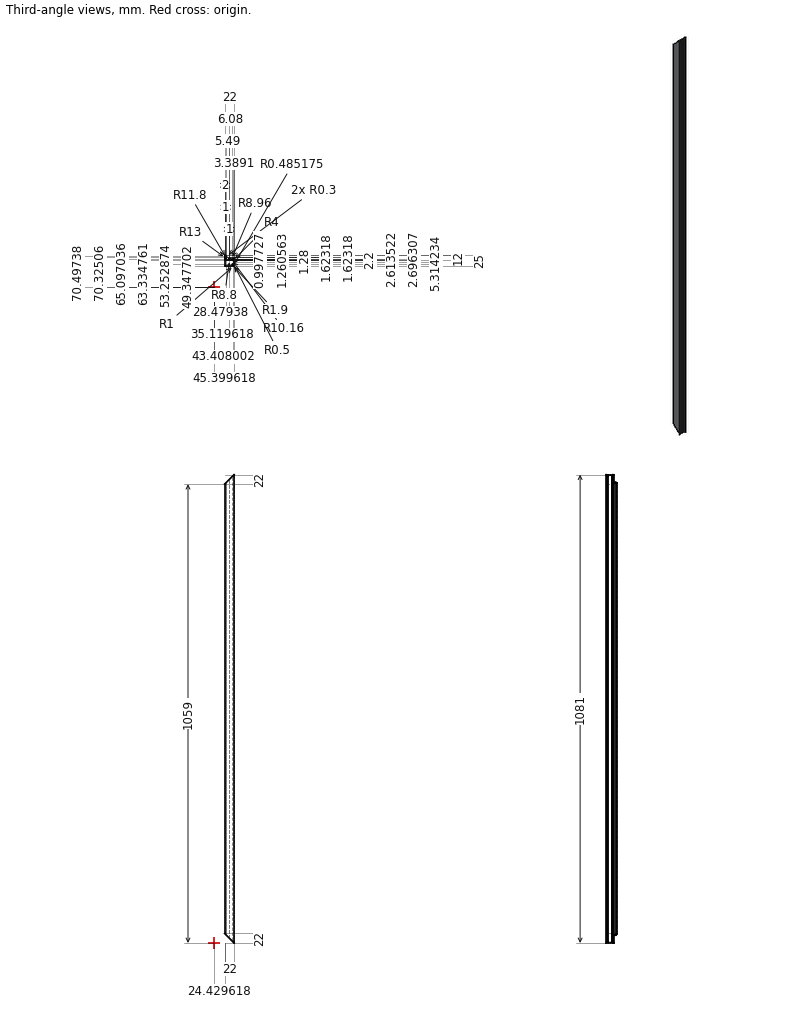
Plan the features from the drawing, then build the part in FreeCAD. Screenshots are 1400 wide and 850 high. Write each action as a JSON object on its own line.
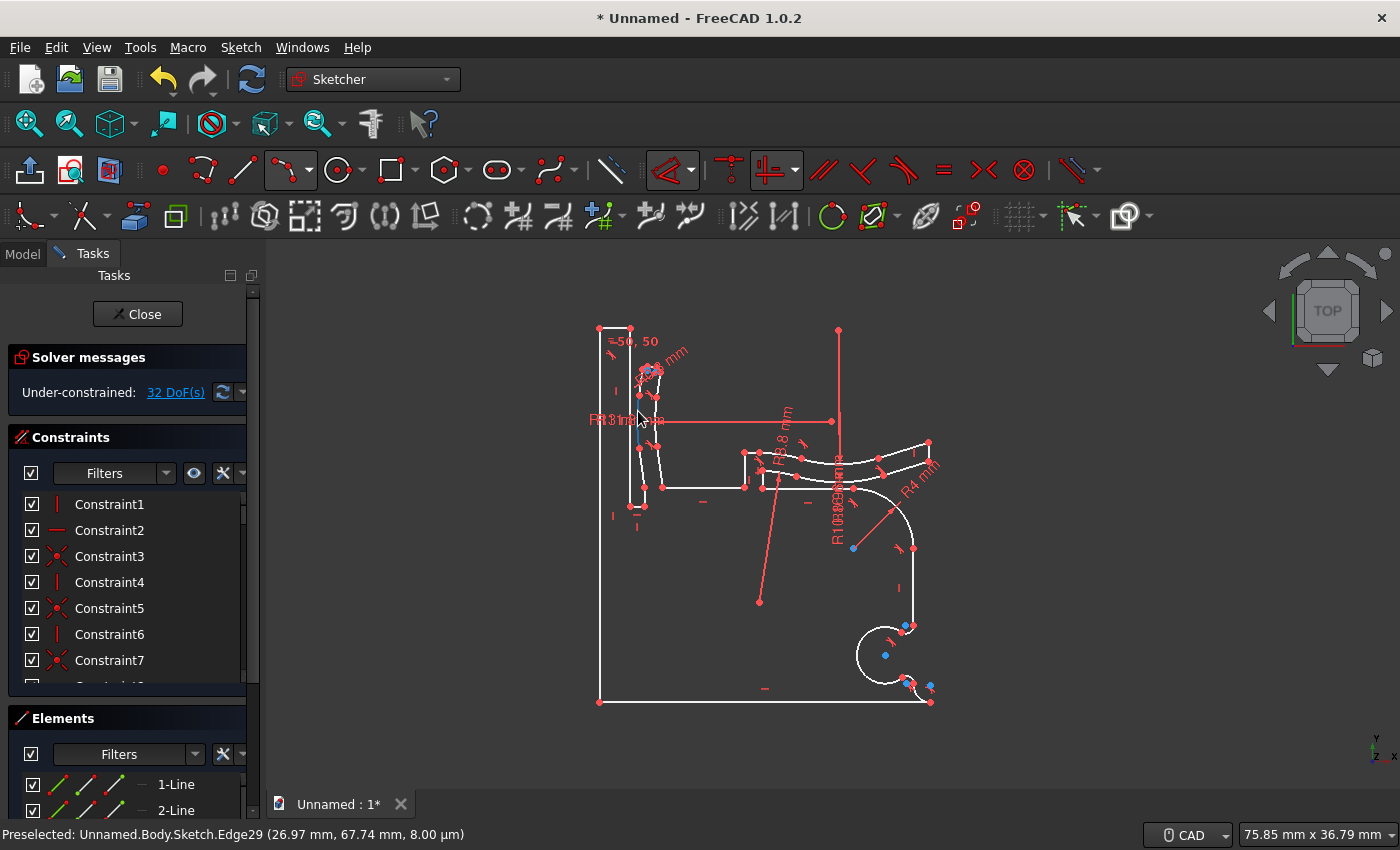
{"action": "scroll", "coordinate": [915, 692], "scroll_direction": "up", "scroll_amount": 5}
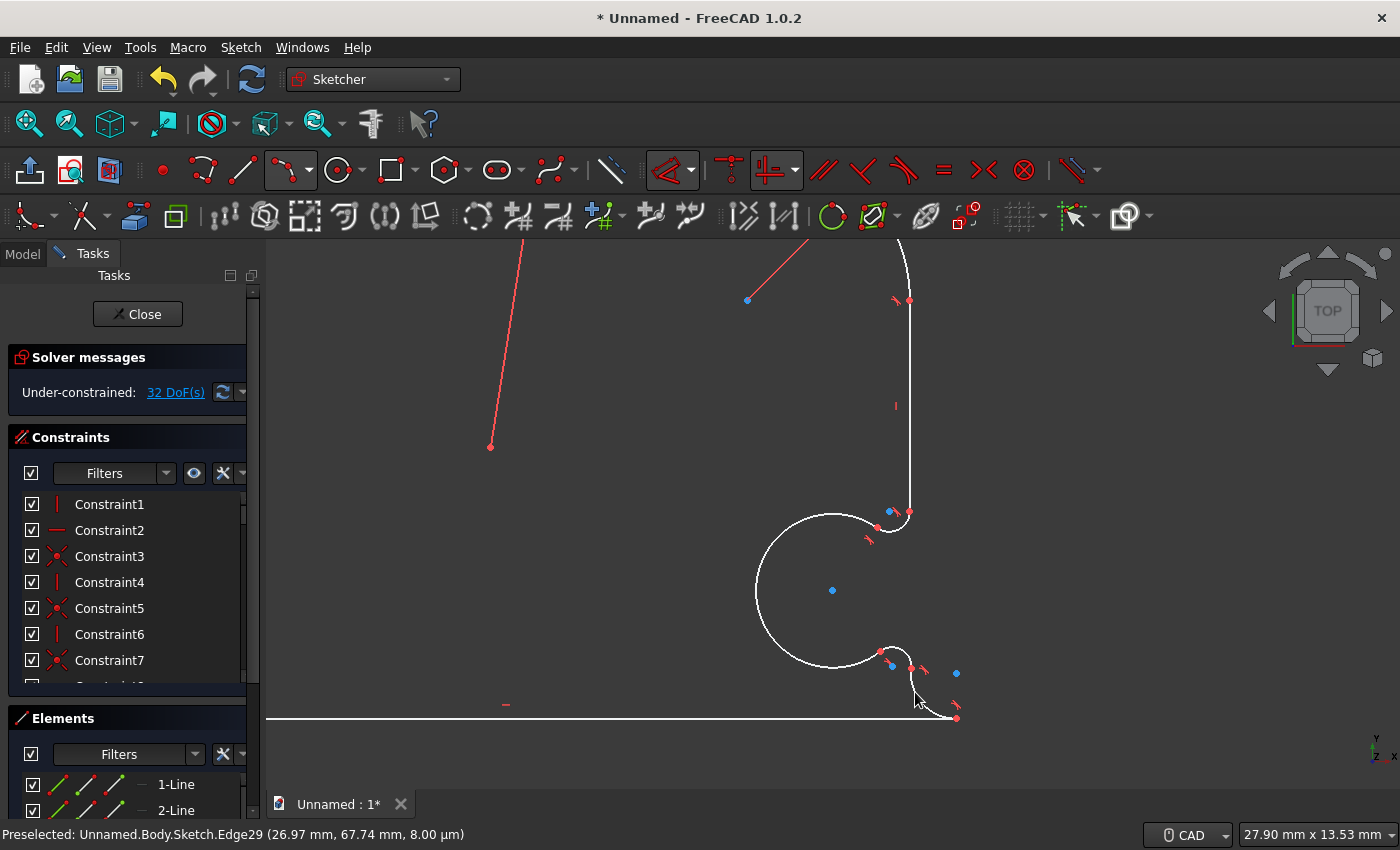
{"action": "left_click", "coordinate": [914, 691]}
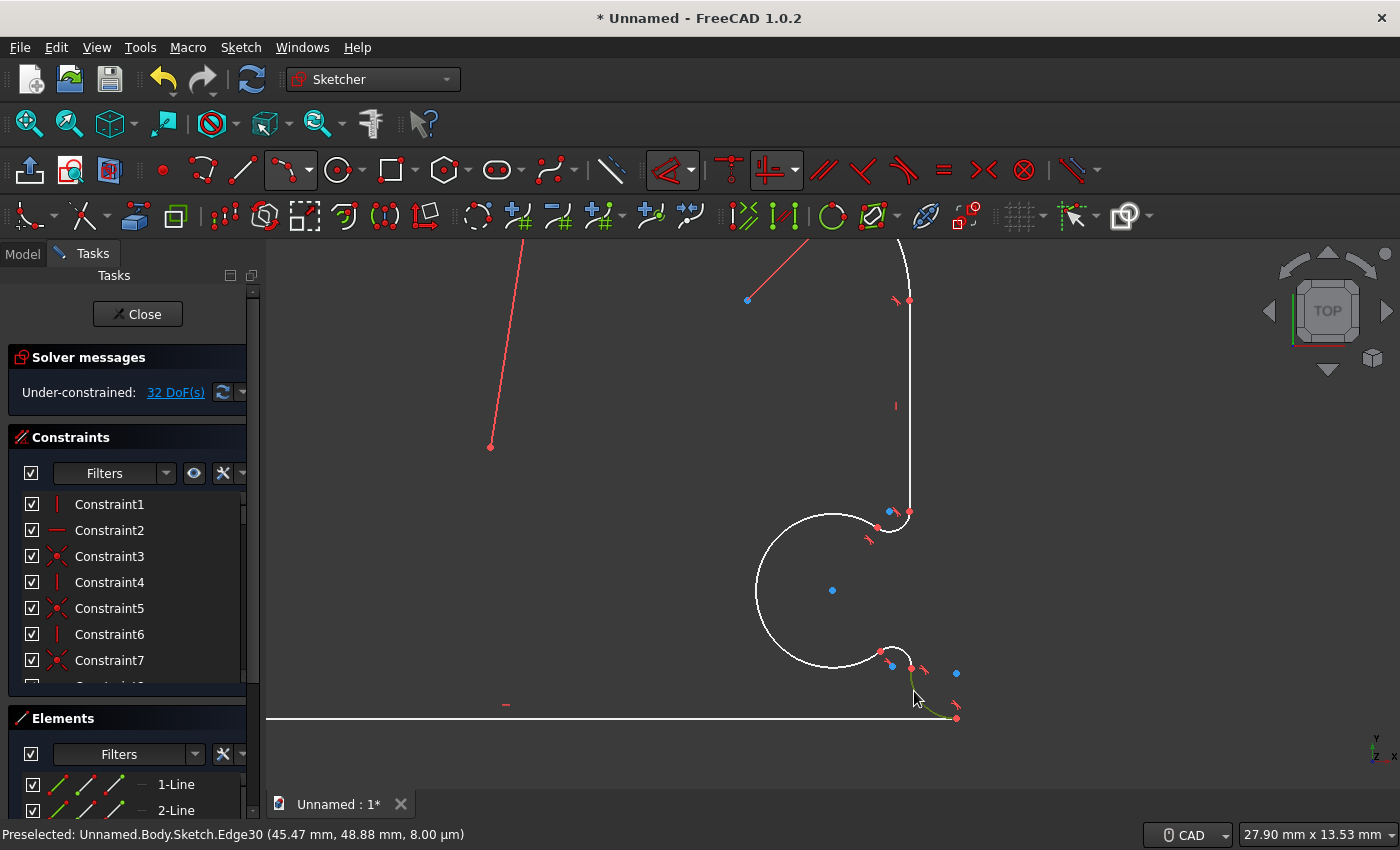
{"action": "left_click", "coordinate": [694, 170]}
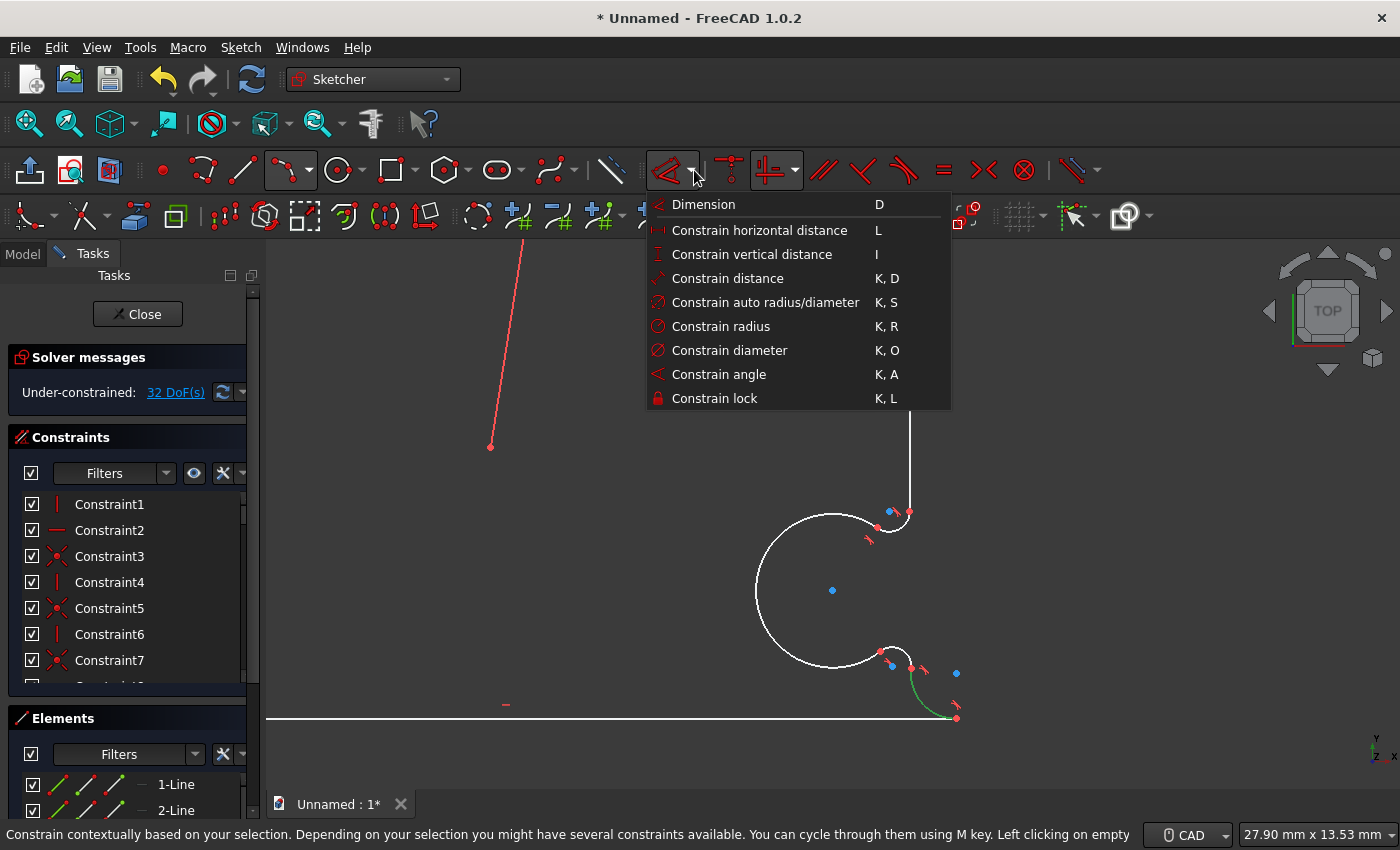
{"action": "left_click", "coordinate": [799, 326]}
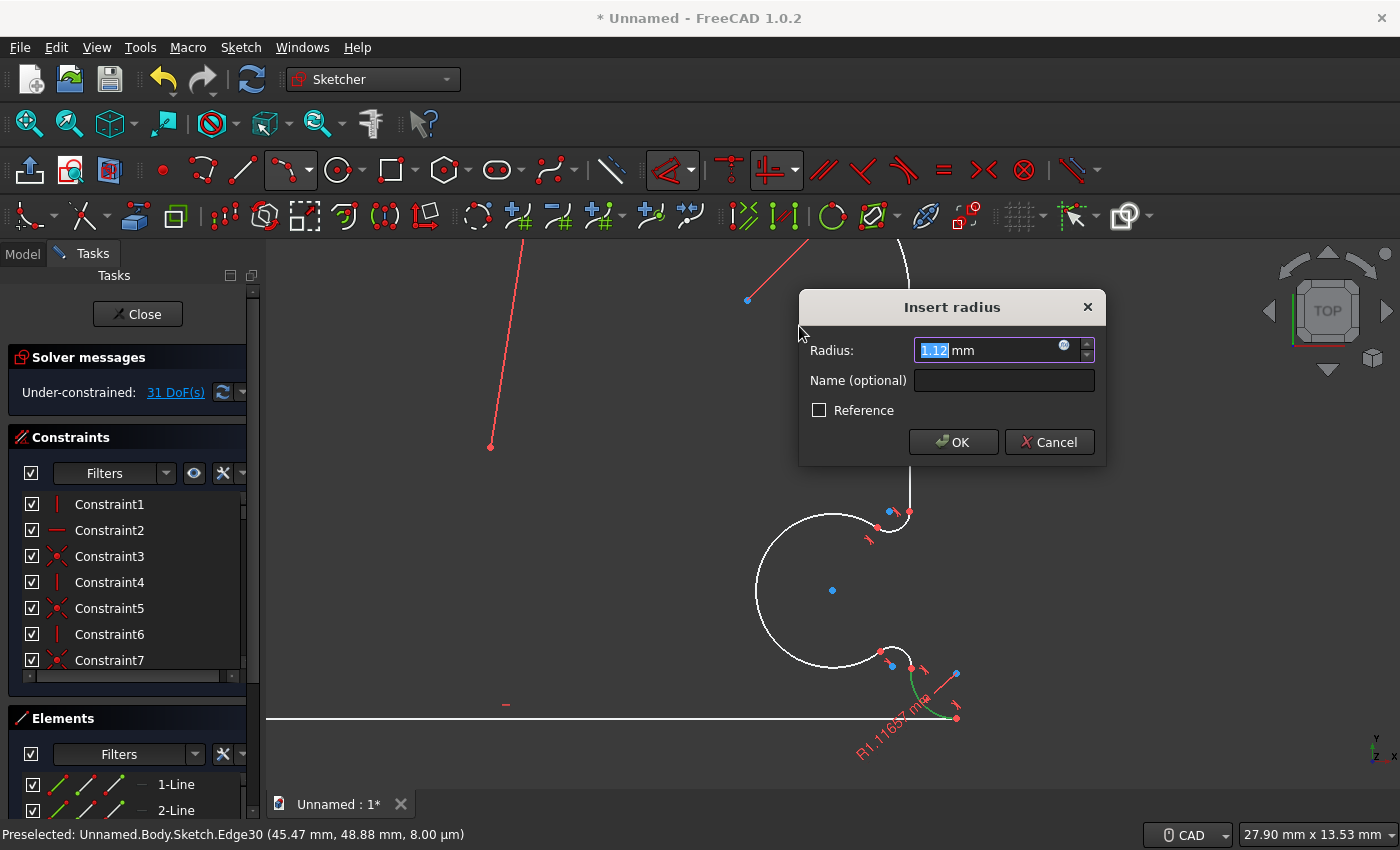
{"action": "type", "text": "1"}
{"action": "key", "text": "Return"}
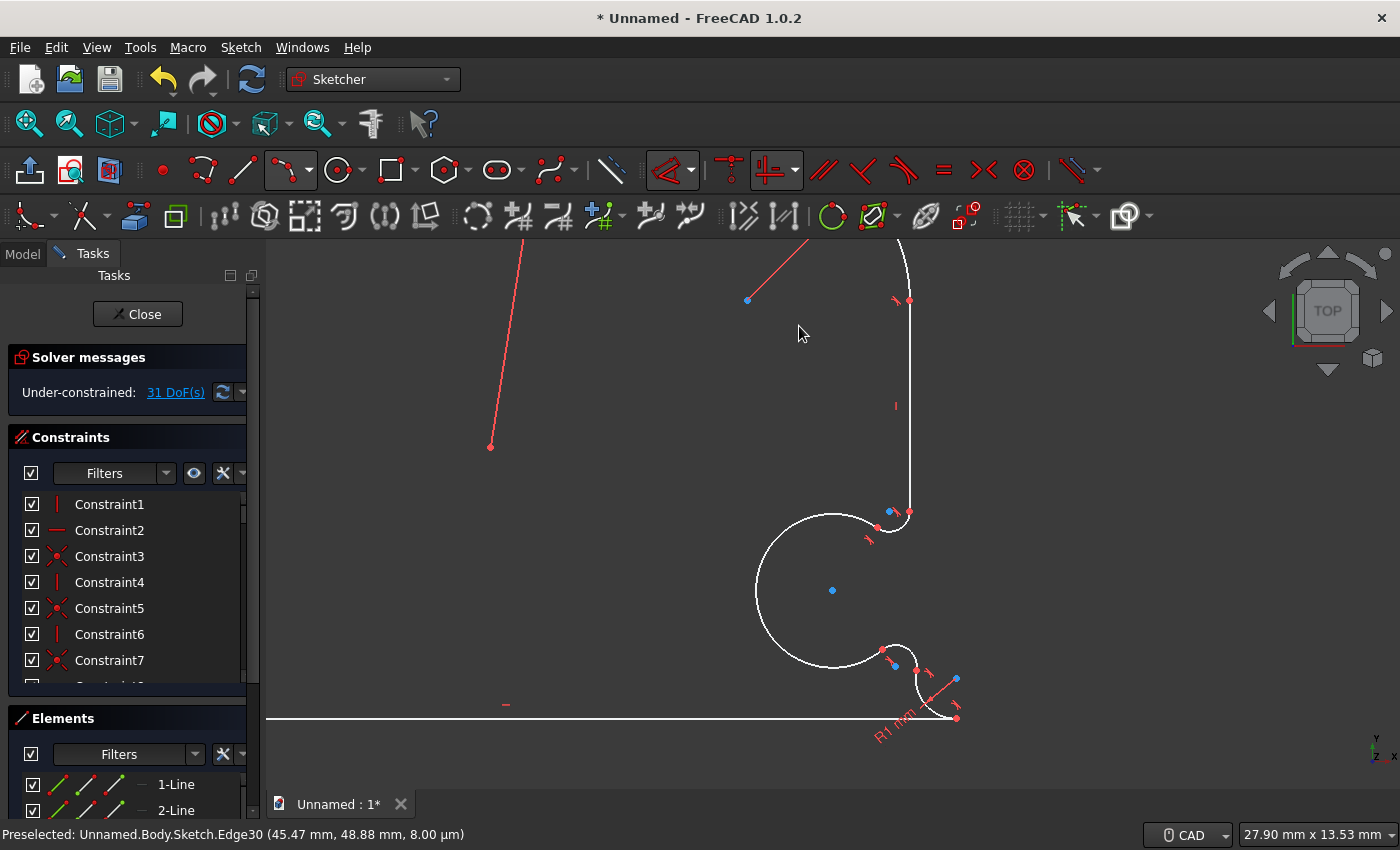
{"action": "scroll", "coordinate": [914, 655], "scroll_direction": "up", "scroll_amount": 4}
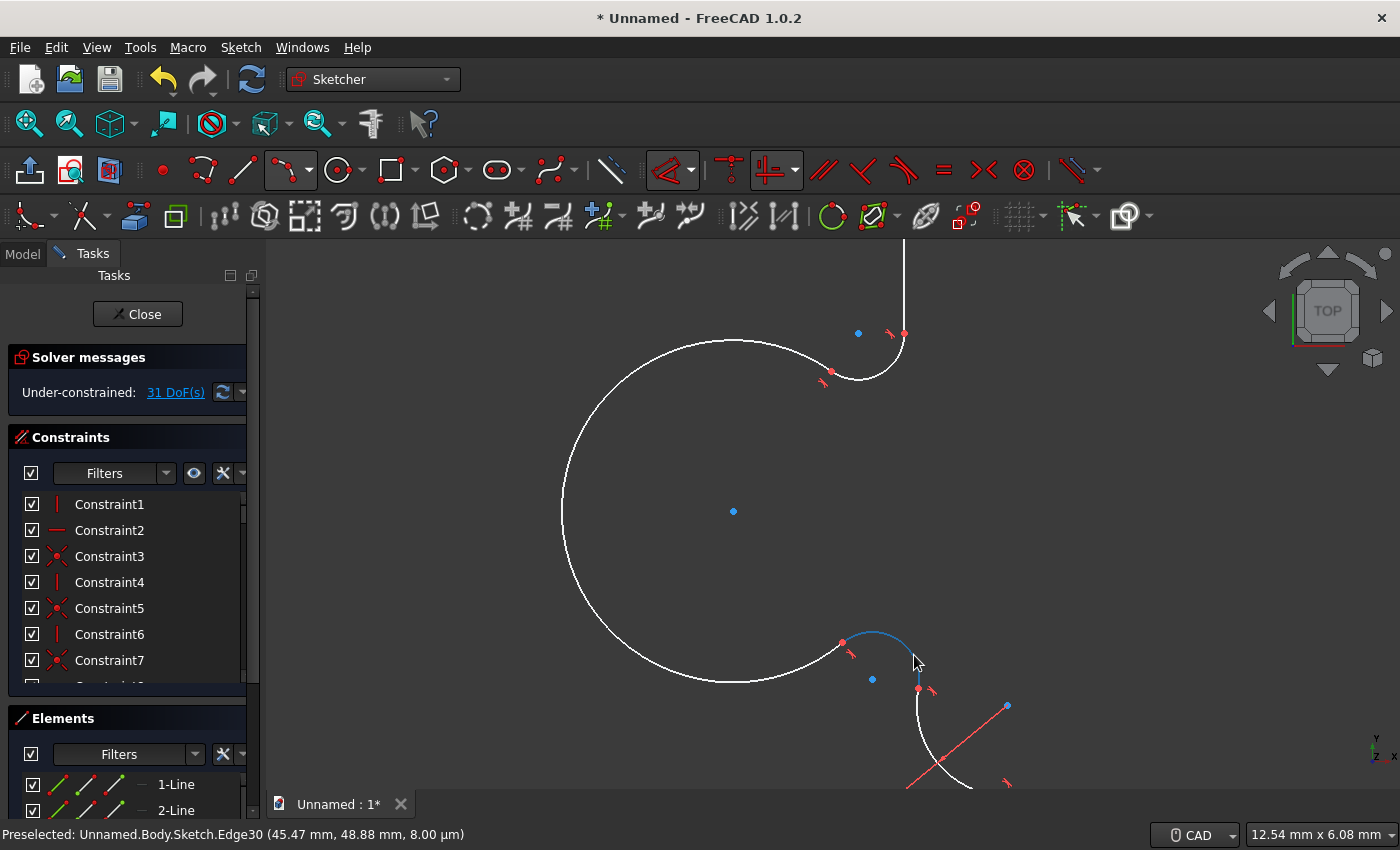
{"action": "left_click", "coordinate": [913, 655]}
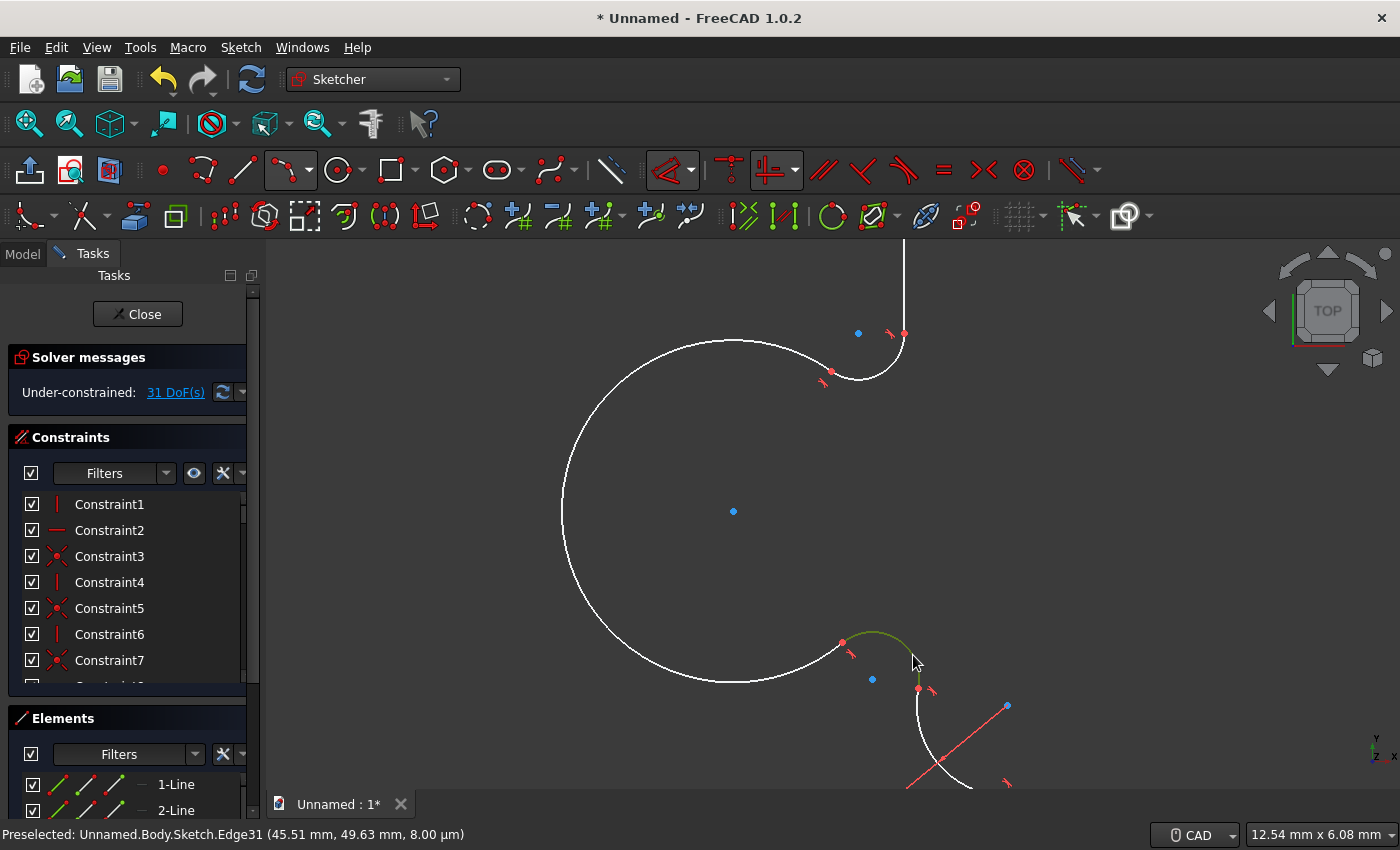
{"action": "key", "text": "k r"}